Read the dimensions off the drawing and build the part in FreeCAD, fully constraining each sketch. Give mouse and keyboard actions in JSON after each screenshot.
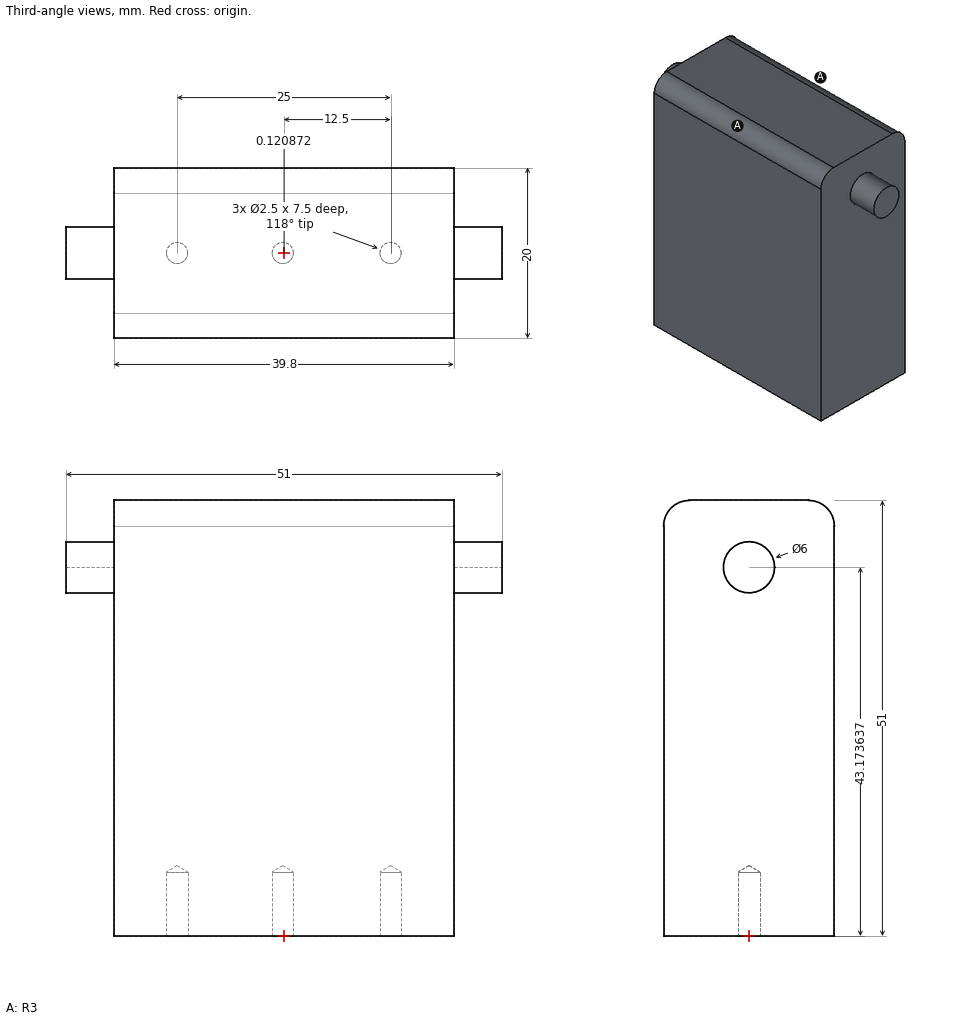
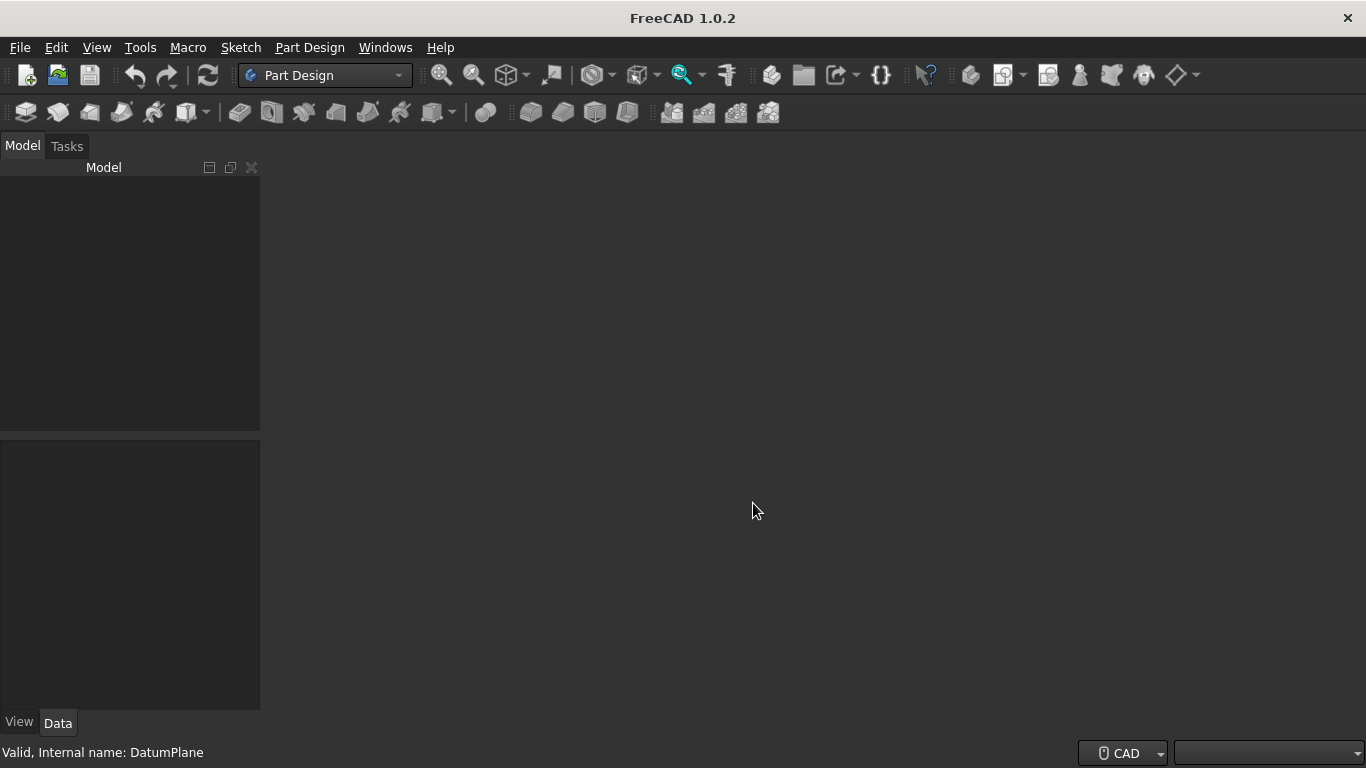
{"action": "key", "text": "ctrl+n"}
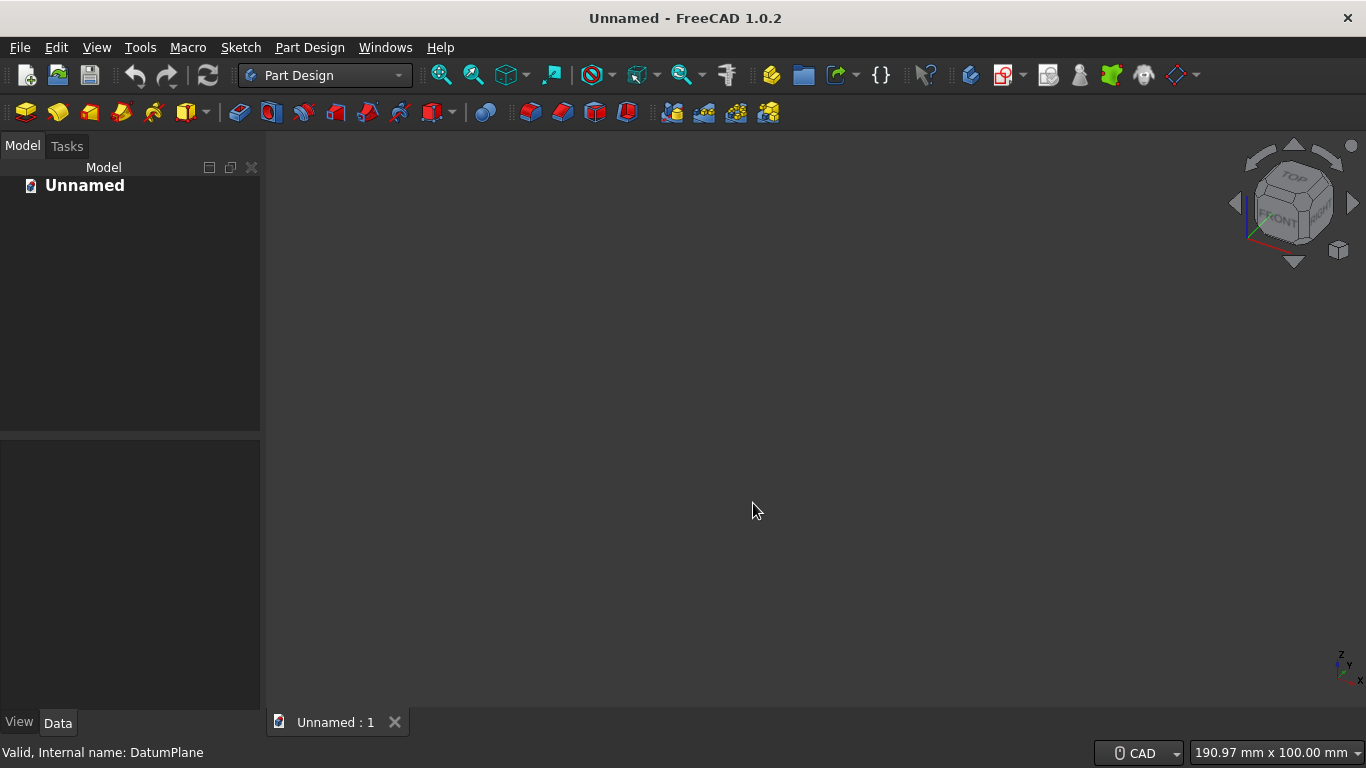
{"action": "left_click", "coordinate": [1004, 76]}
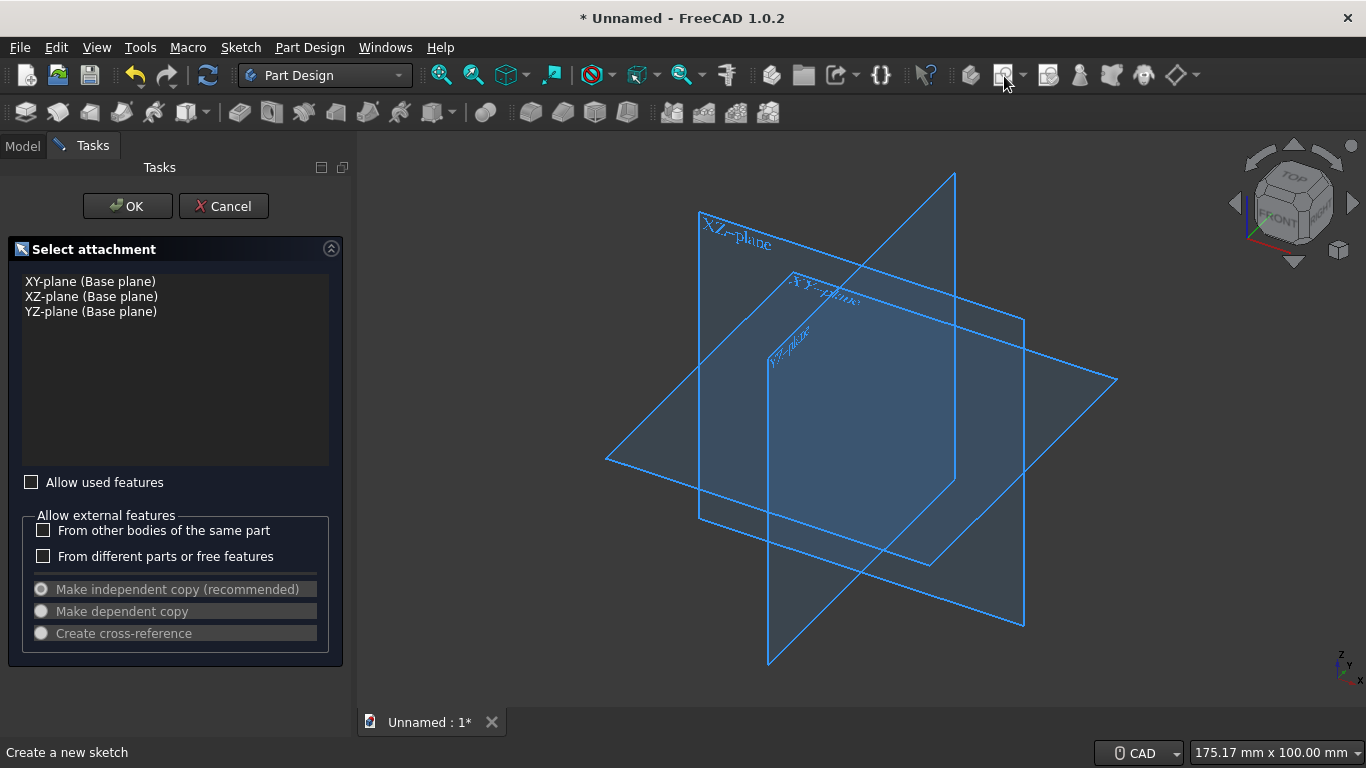
{"action": "left_click", "coordinate": [82, 282]}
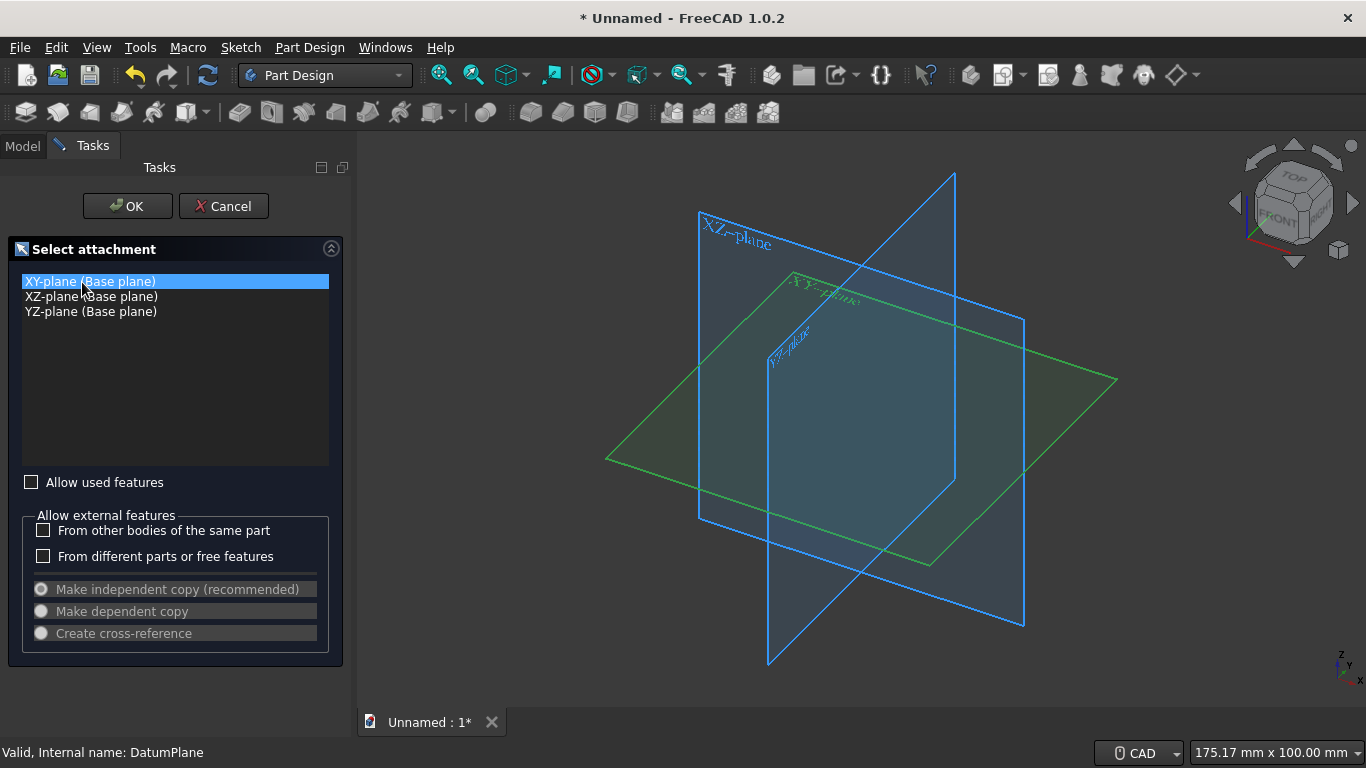
{"action": "left_click", "coordinate": [128, 206]}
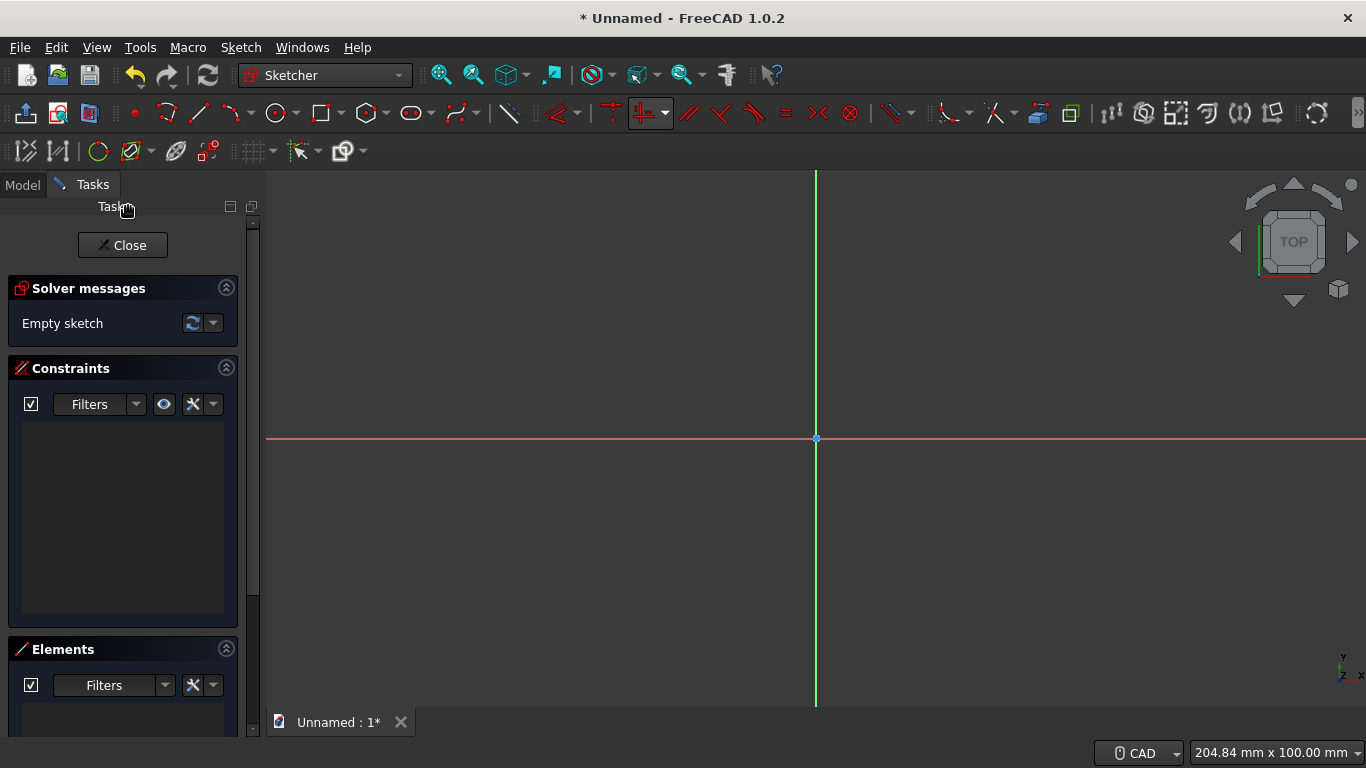
{"action": "scroll", "coordinate": [856, 439], "scroll_direction": "up", "scroll_amount": 5}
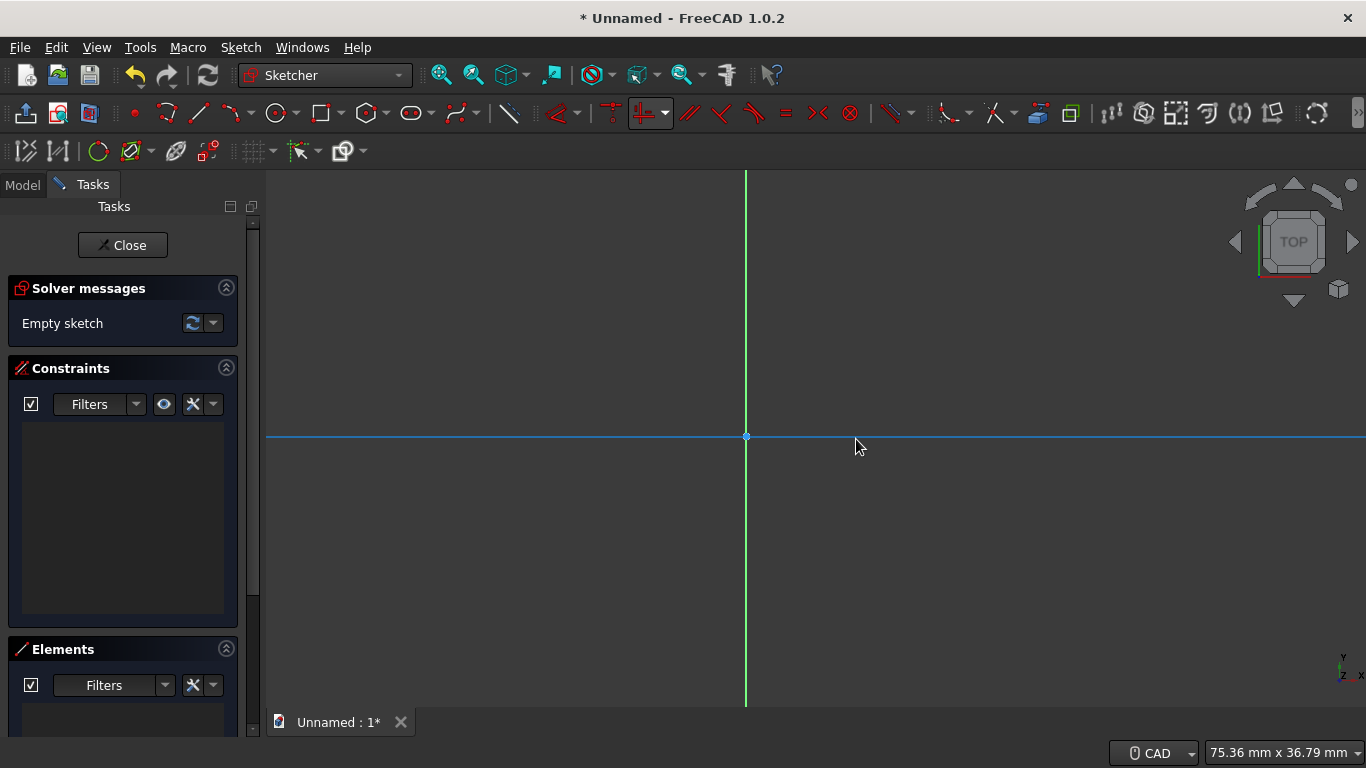
{"action": "key", "text": "g v"}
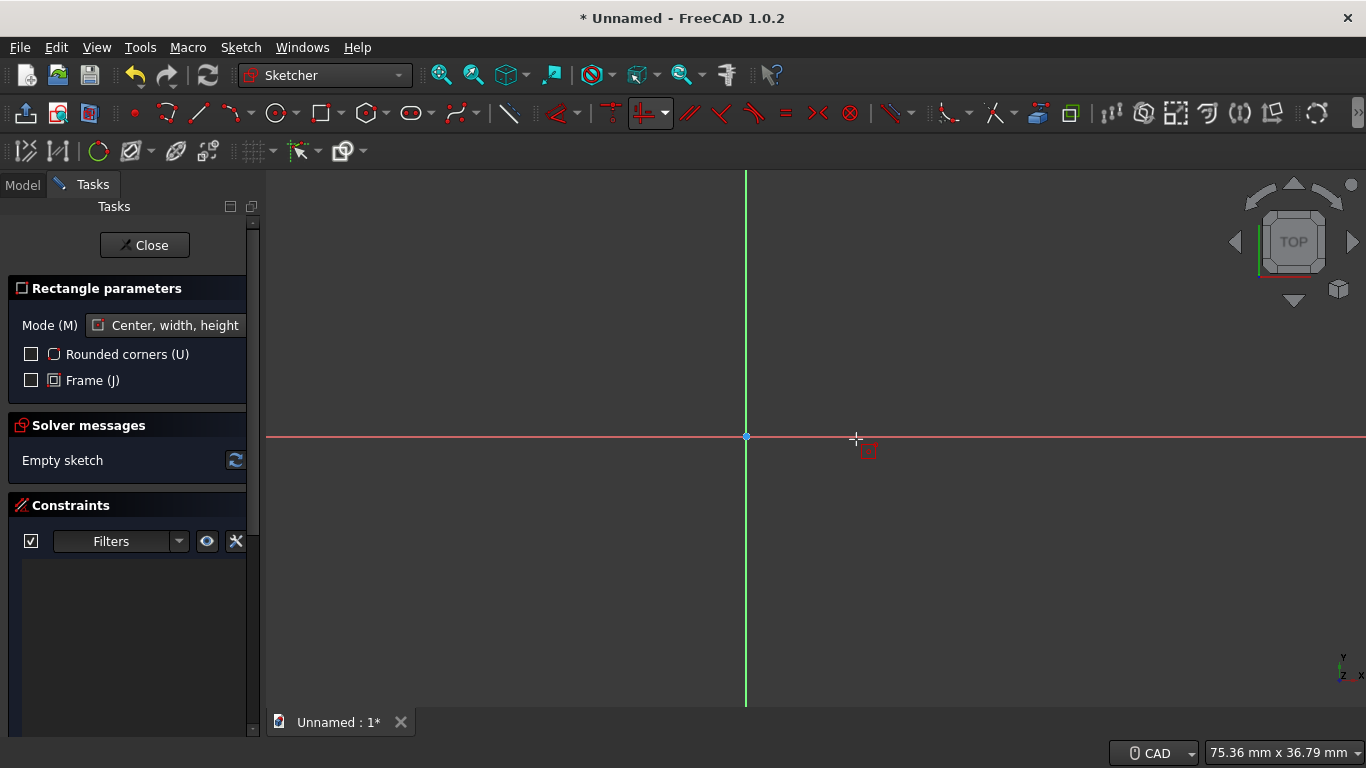
{"action": "left_click", "coordinate": [746, 437]}
{"action": "left_click", "coordinate": [1037, 291]}
{"action": "key", "text": "Escape"}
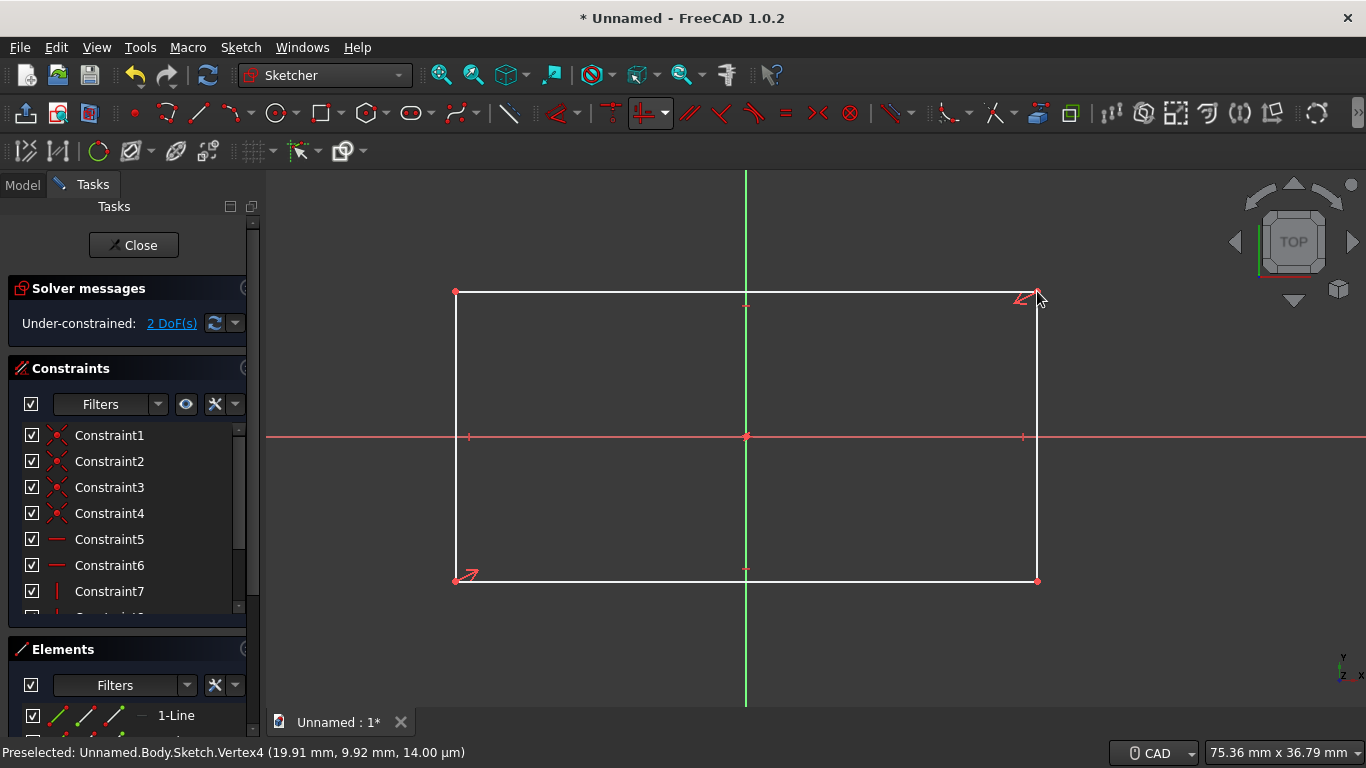
{"action": "left_click", "coordinate": [1037, 495]}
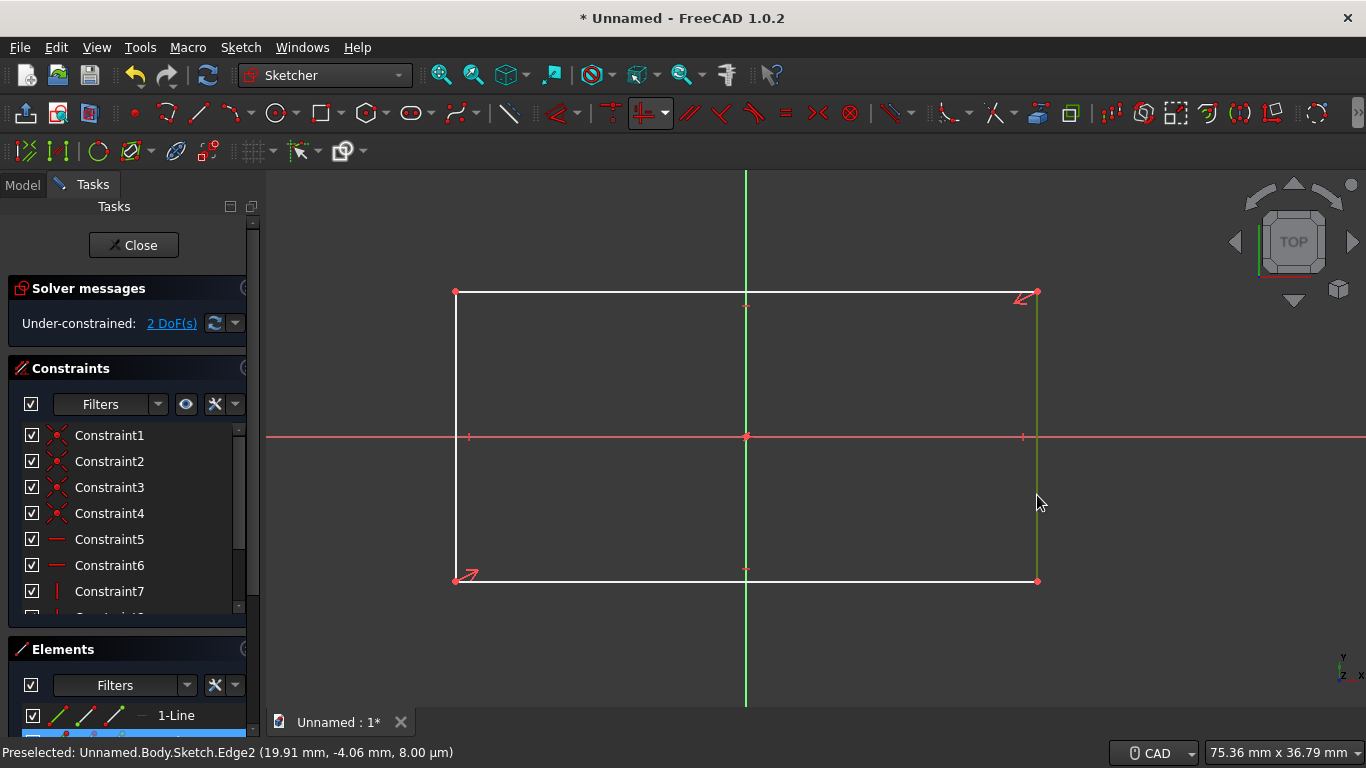
{"action": "left_click", "coordinate": [580, 114]}